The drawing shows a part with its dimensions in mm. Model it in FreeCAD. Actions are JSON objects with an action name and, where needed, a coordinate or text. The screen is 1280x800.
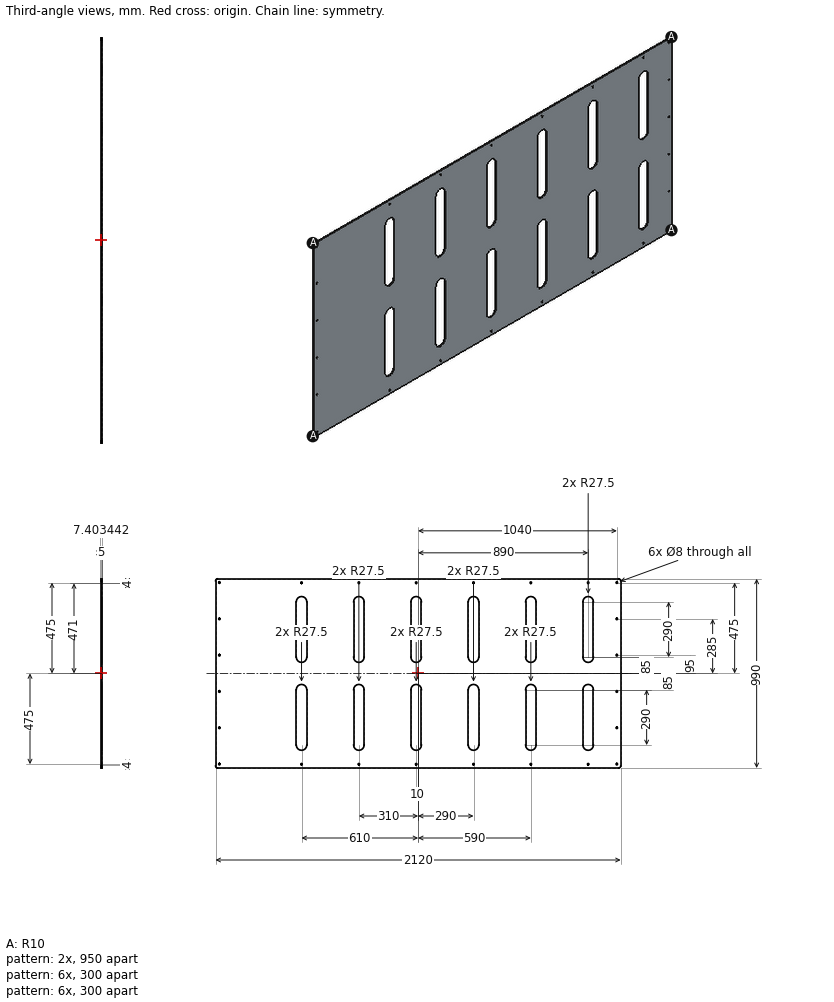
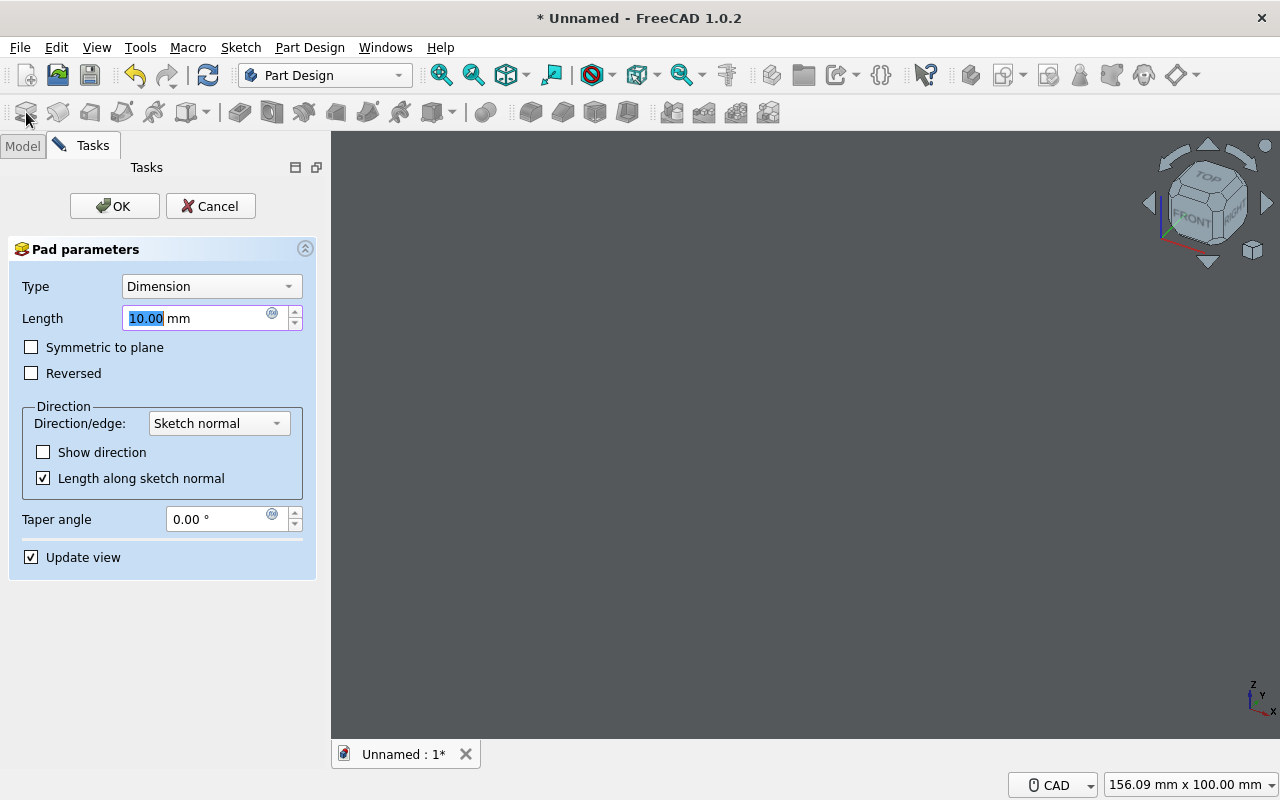
{"action": "type", "text": "5"}
{"action": "key", "text": "Tab"}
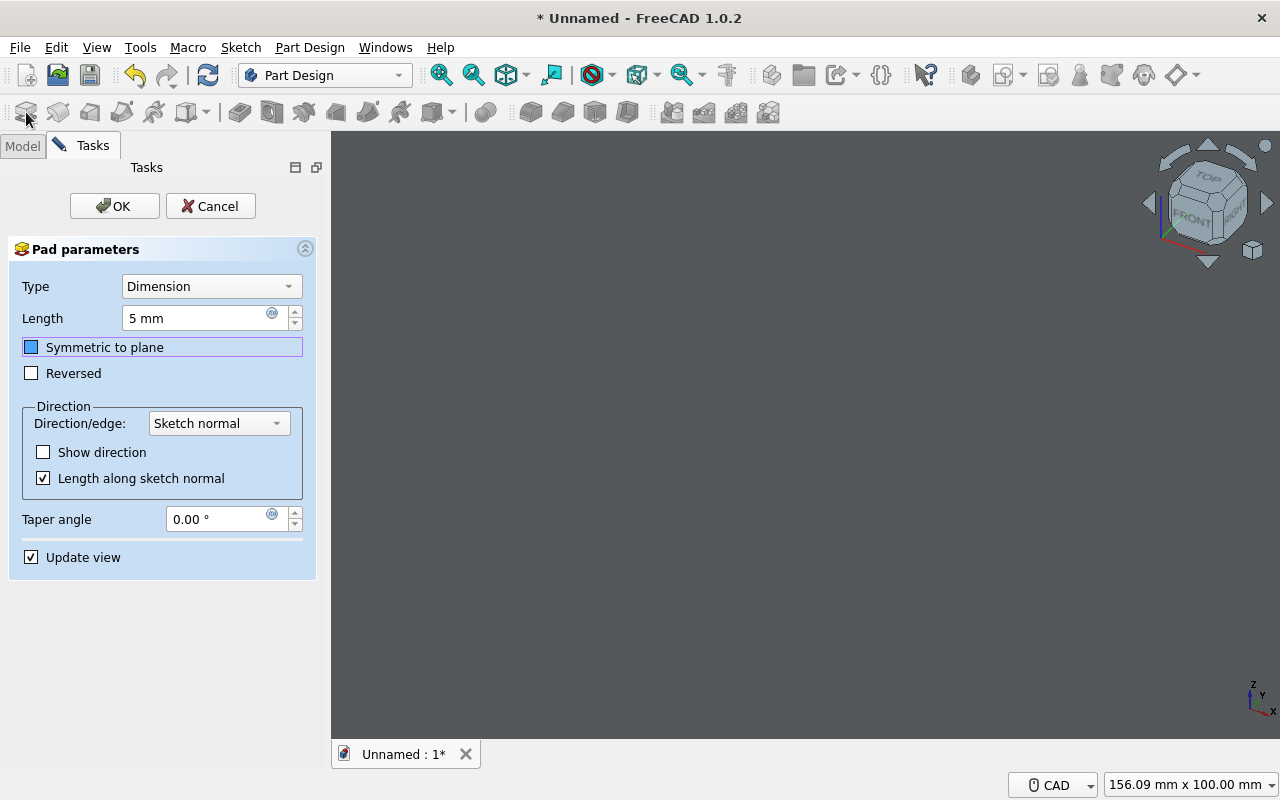
{"action": "left_click", "coordinate": [115, 206]}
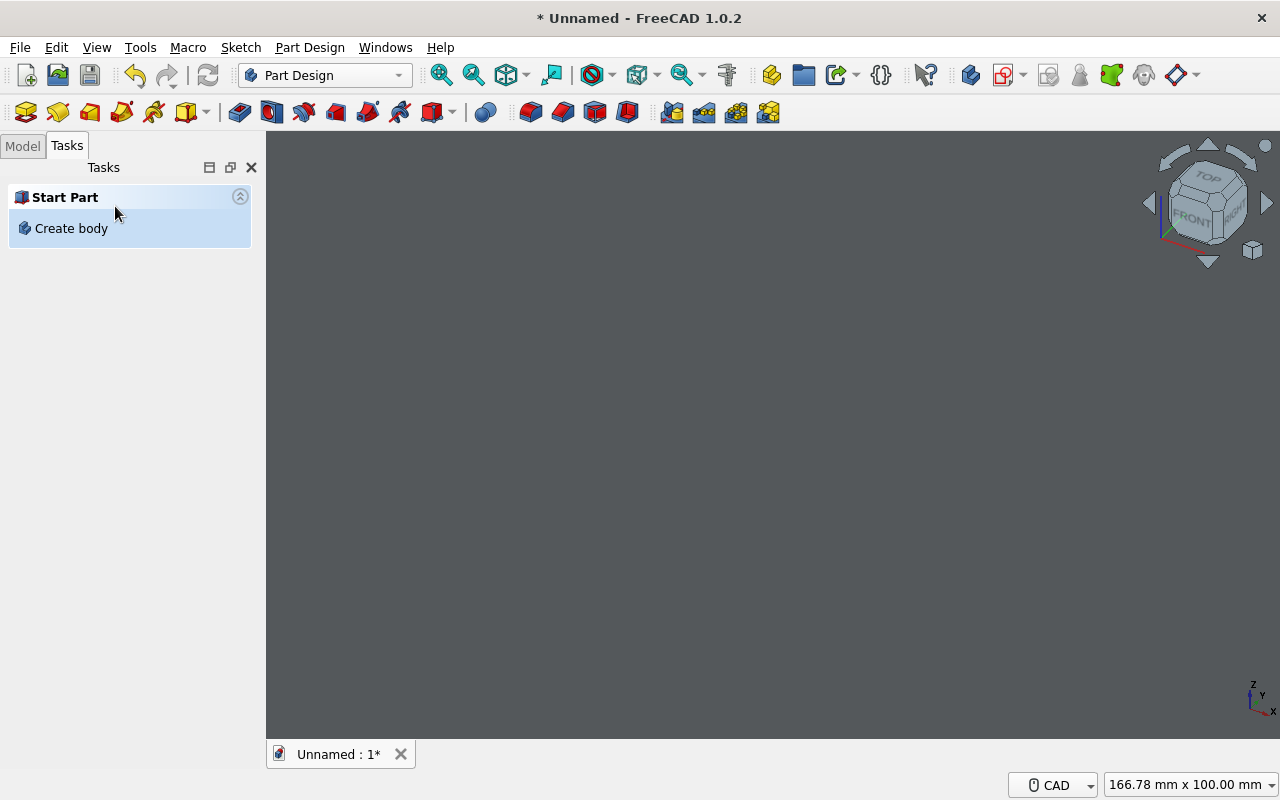
{"action": "left_click", "coordinate": [442, 76]}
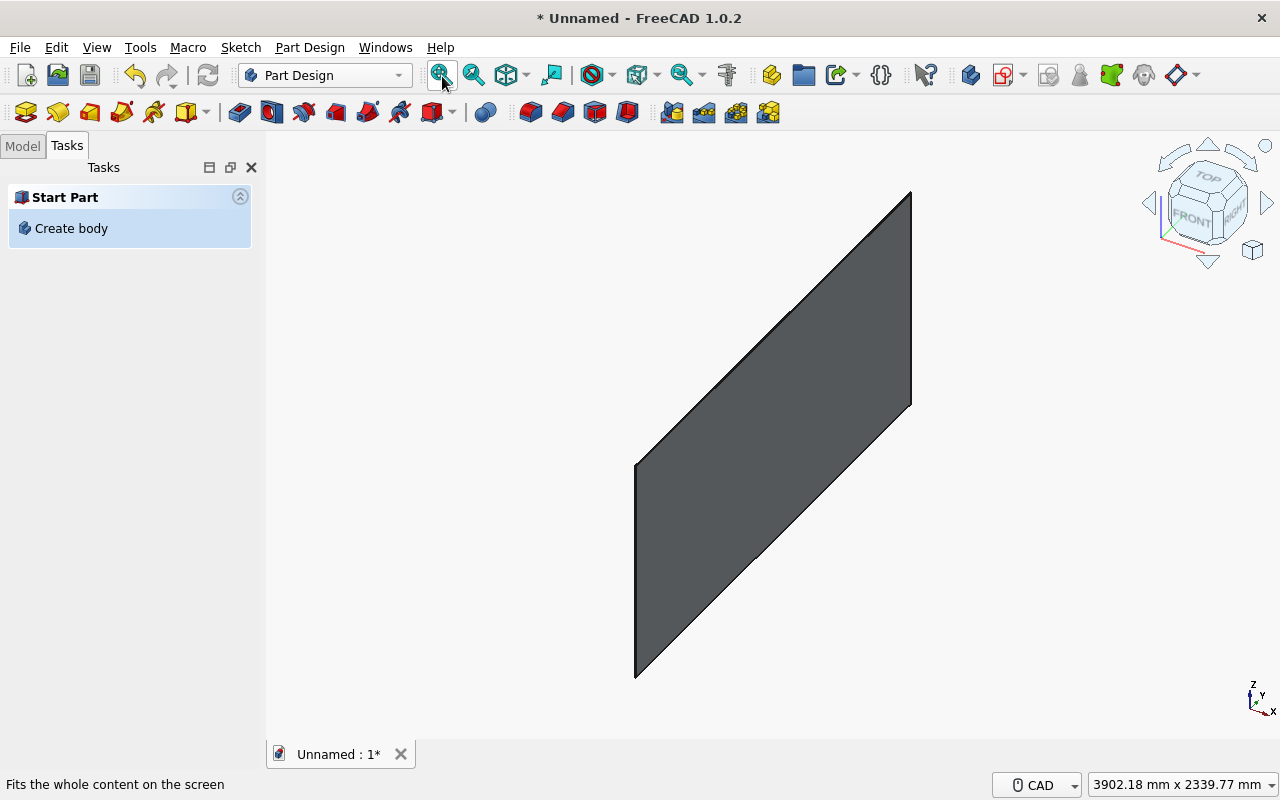
{"action": "scroll", "coordinate": [635, 676], "scroll_direction": "up", "scroll_amount": 15}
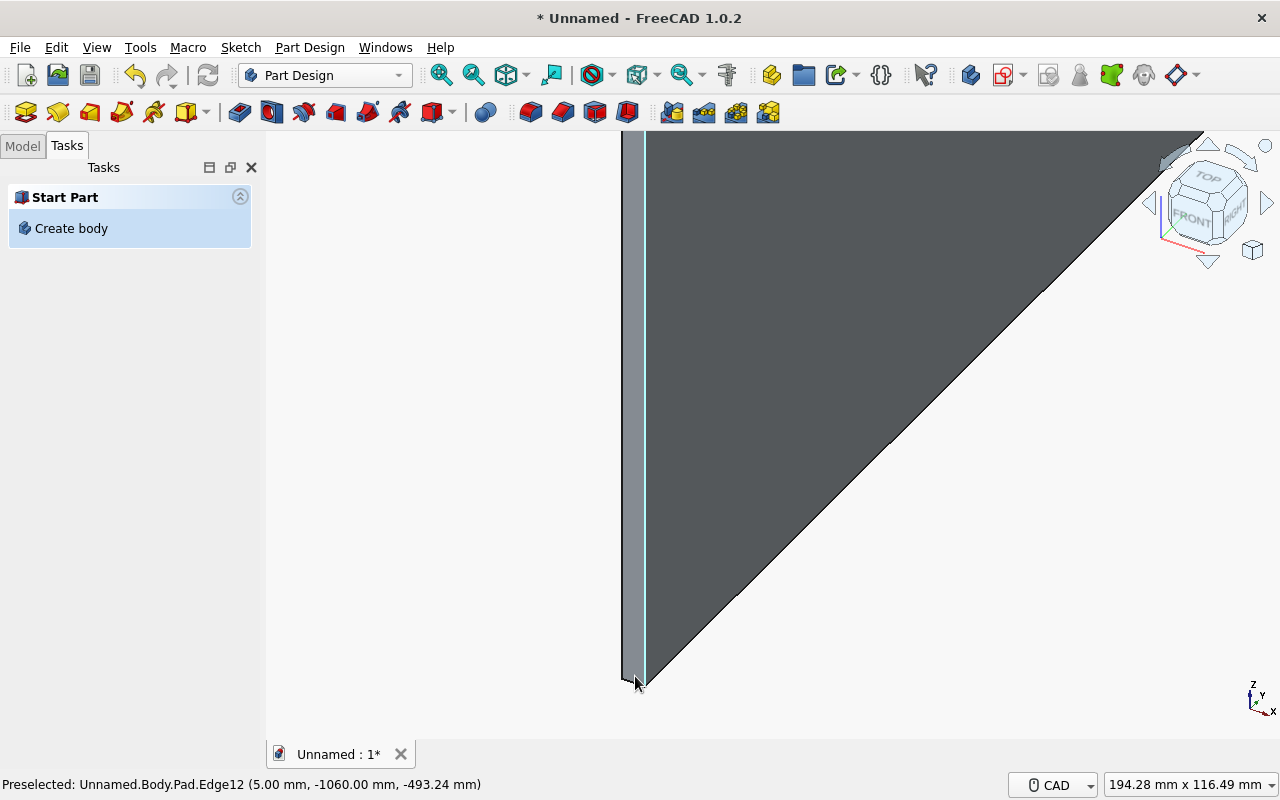
{"action": "left_click", "coordinate": [442, 76]}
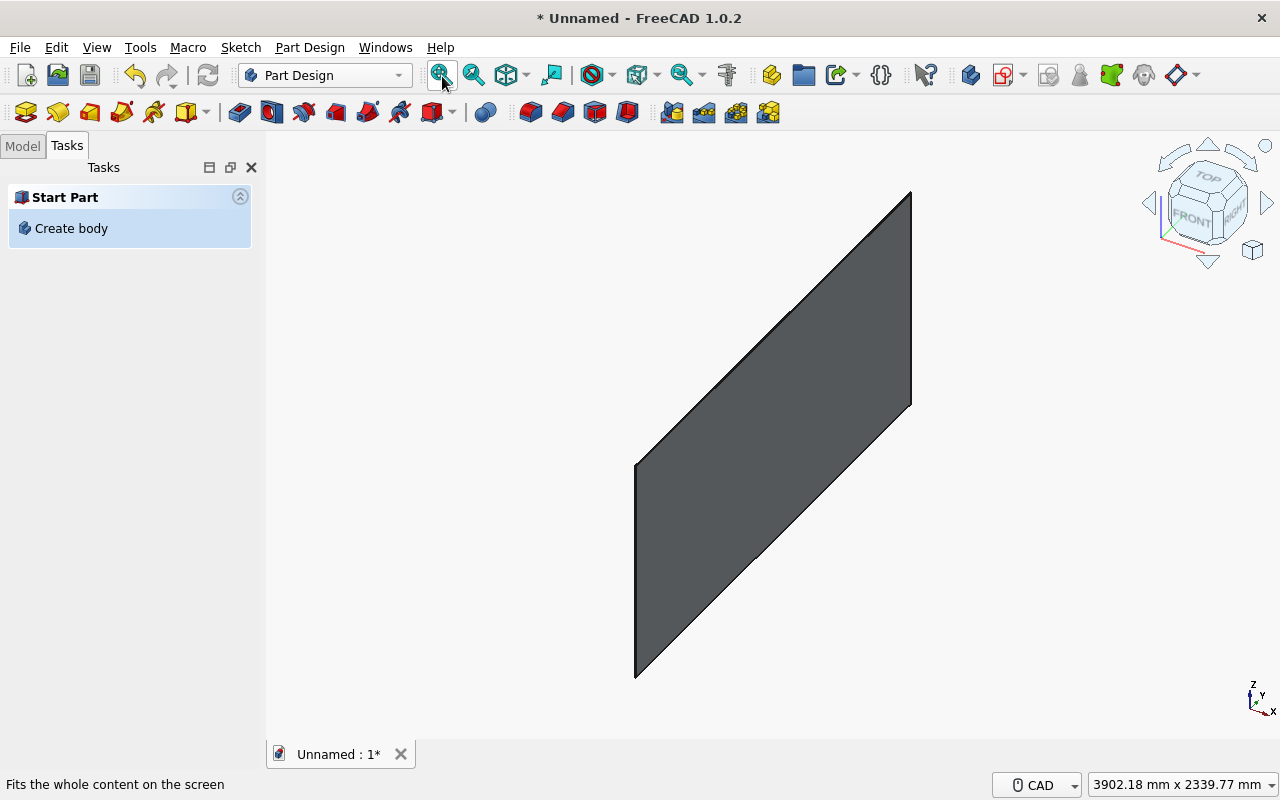
{"action": "key", "text": "0"}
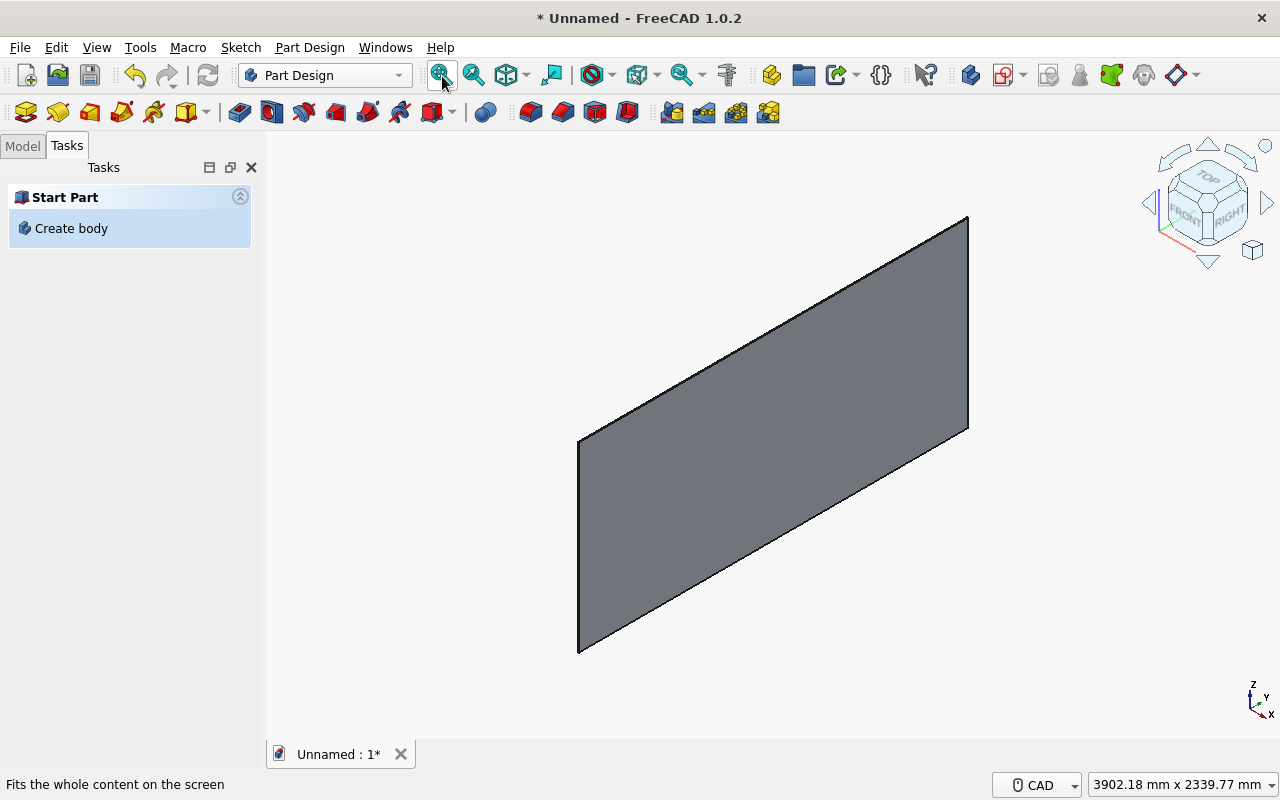
{"action": "scroll", "coordinate": [578, 651], "scroll_direction": "up", "scroll_amount": 15}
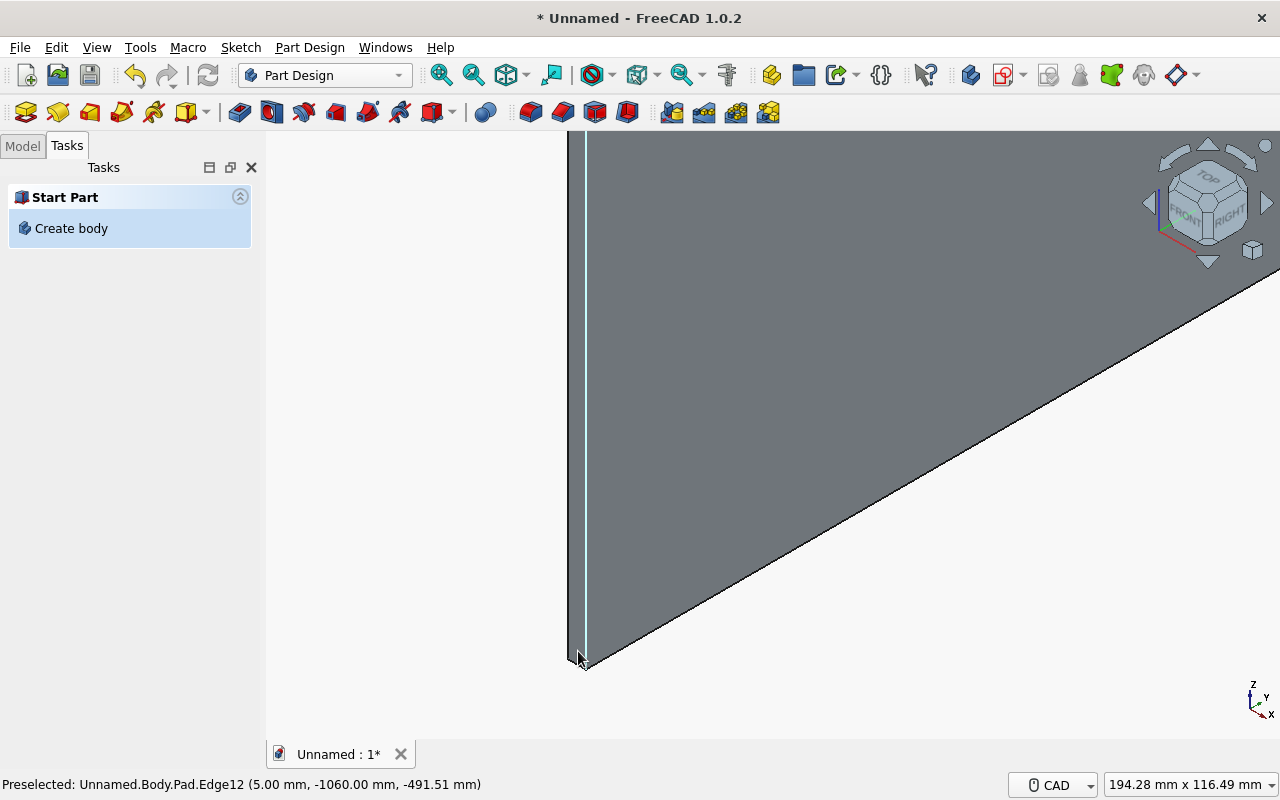
{"action": "left_click", "coordinate": [442, 76]}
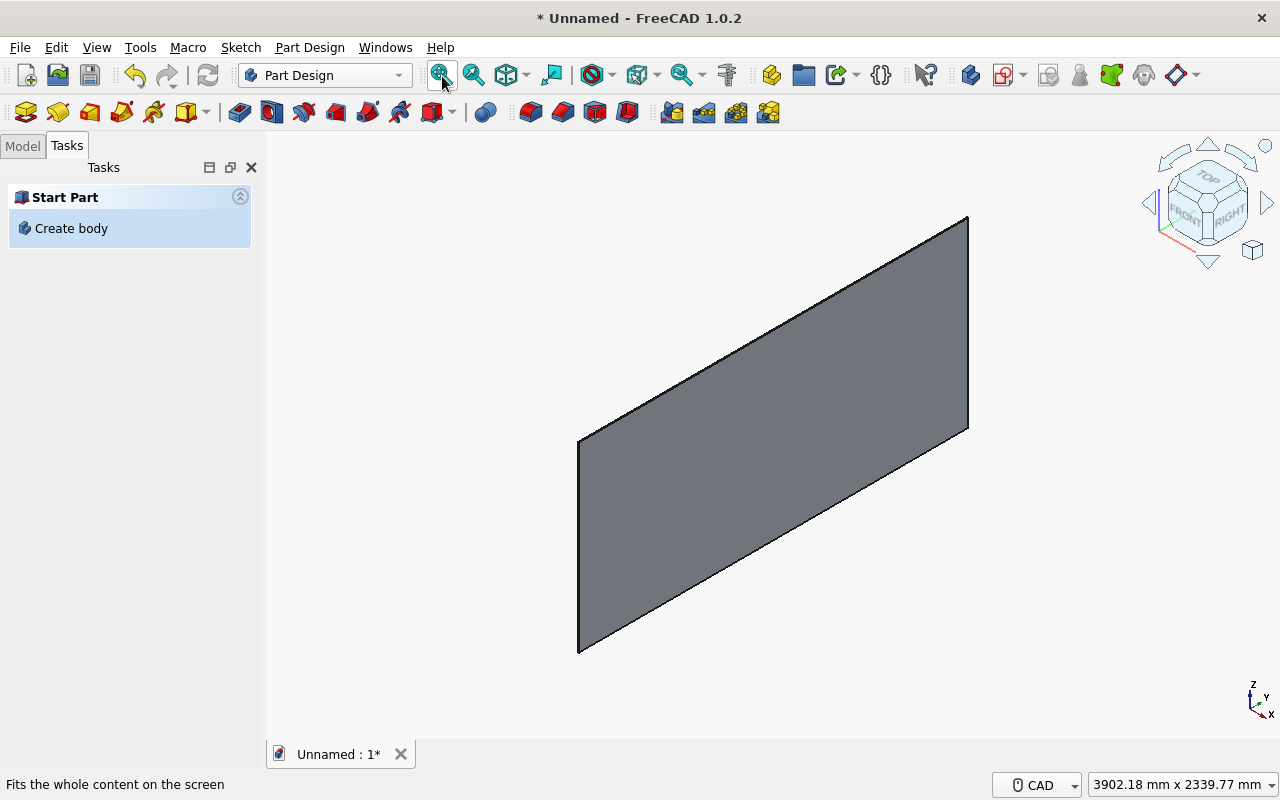
{"action": "key", "text": "2"}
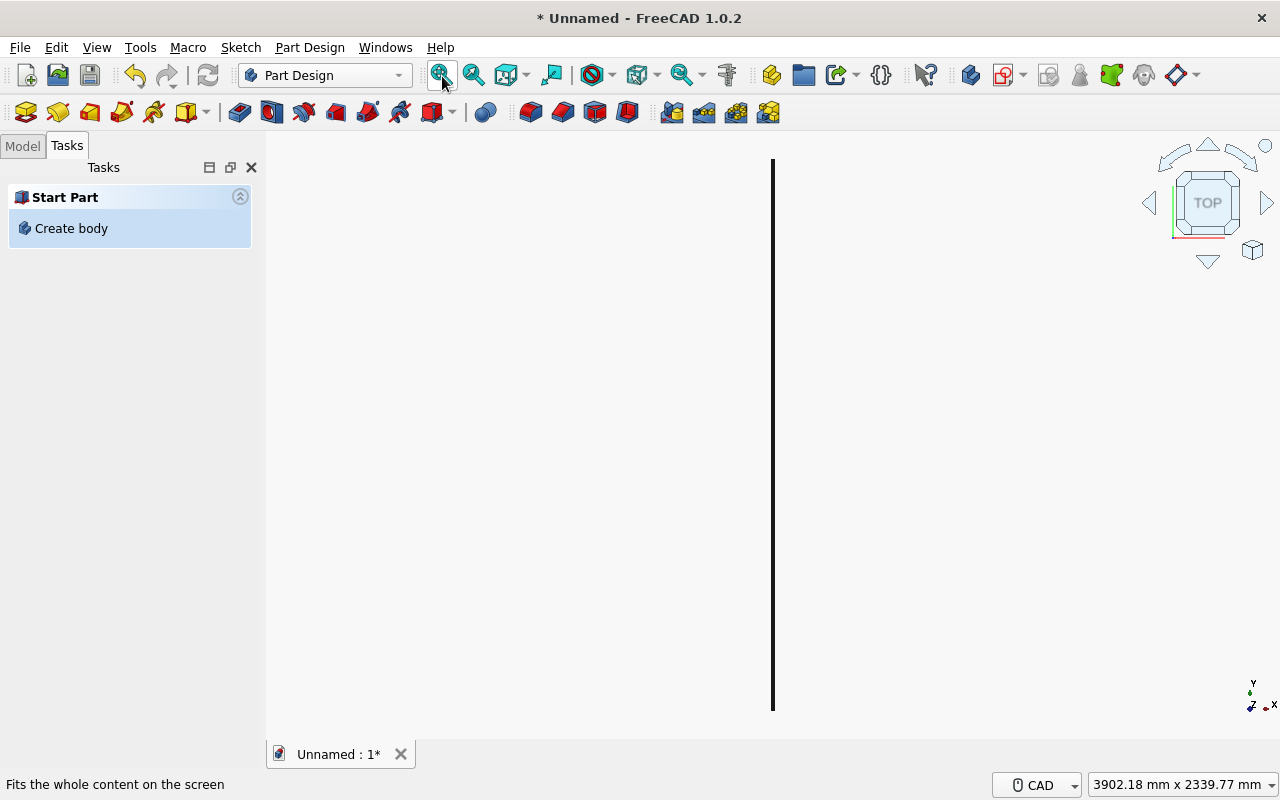
{"action": "scroll", "coordinate": [773, 709], "scroll_direction": "up", "scroll_amount": 15}